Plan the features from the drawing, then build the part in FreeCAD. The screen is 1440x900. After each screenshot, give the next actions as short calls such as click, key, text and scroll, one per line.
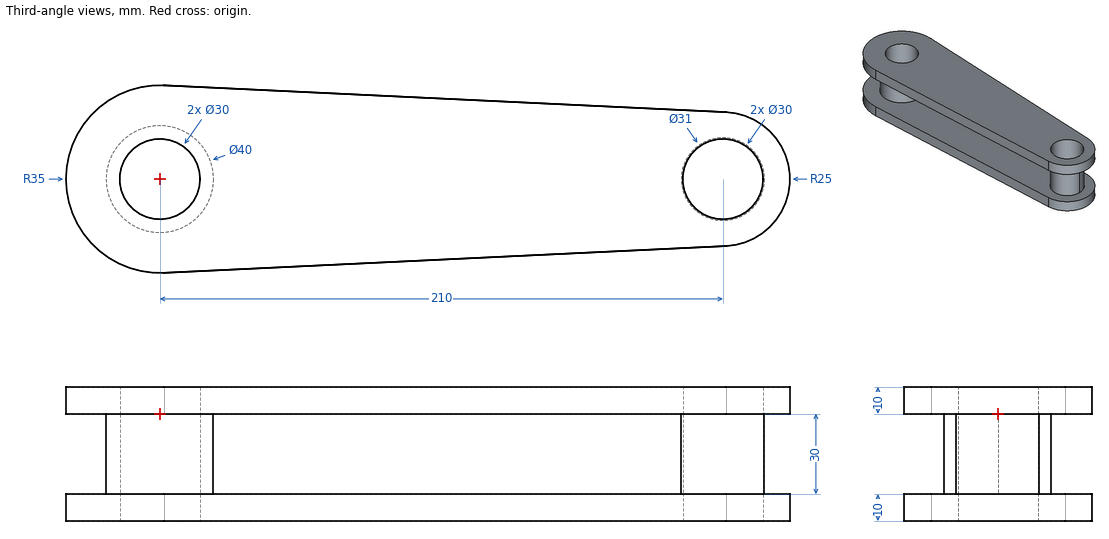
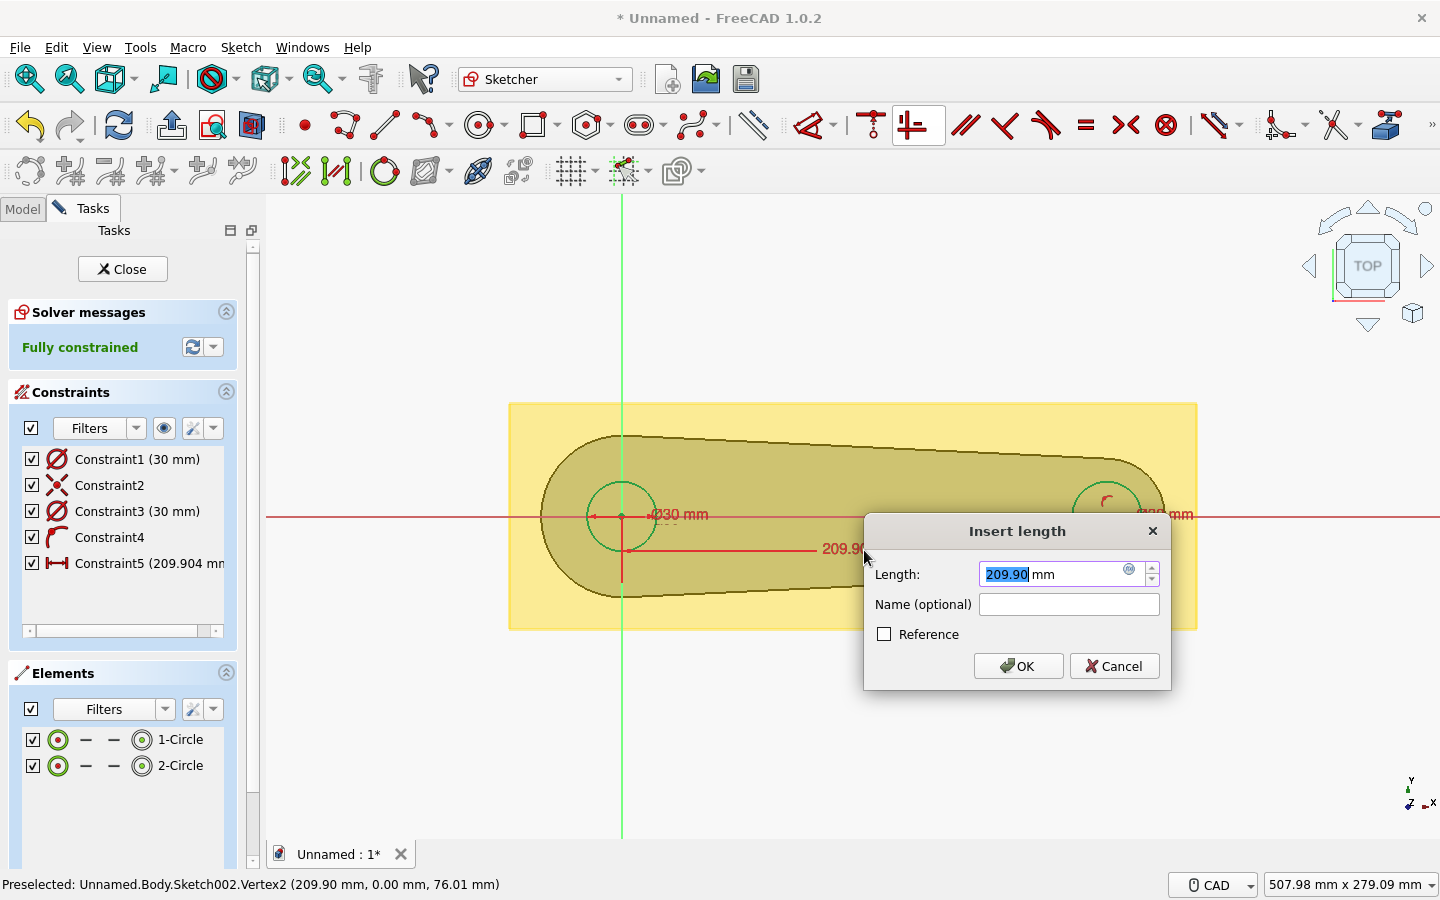
text(210)
key(Return)
key(Escape)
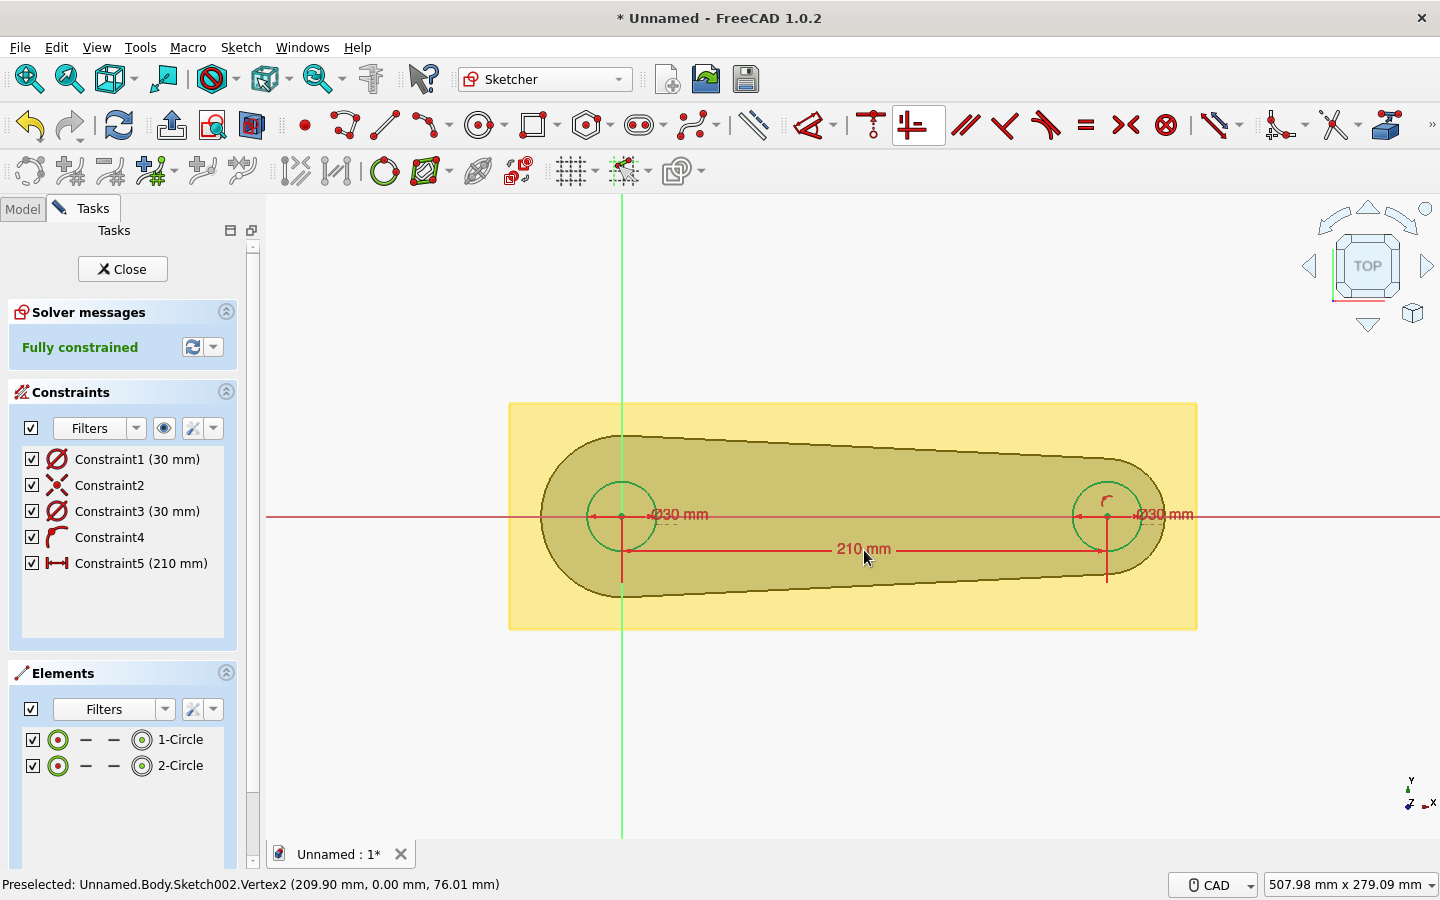
click(123, 269)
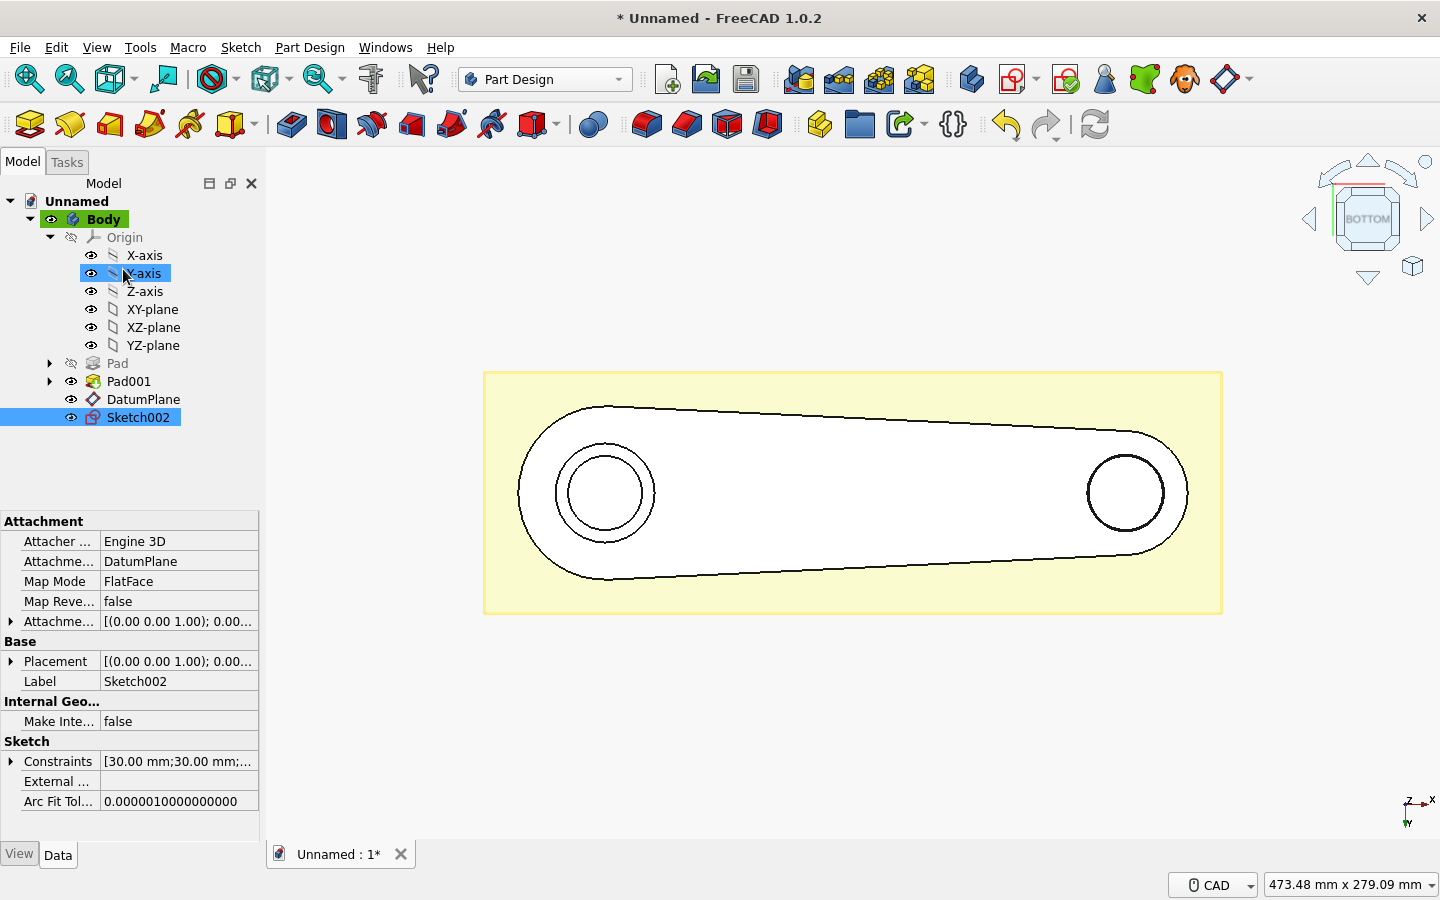
click(292, 124)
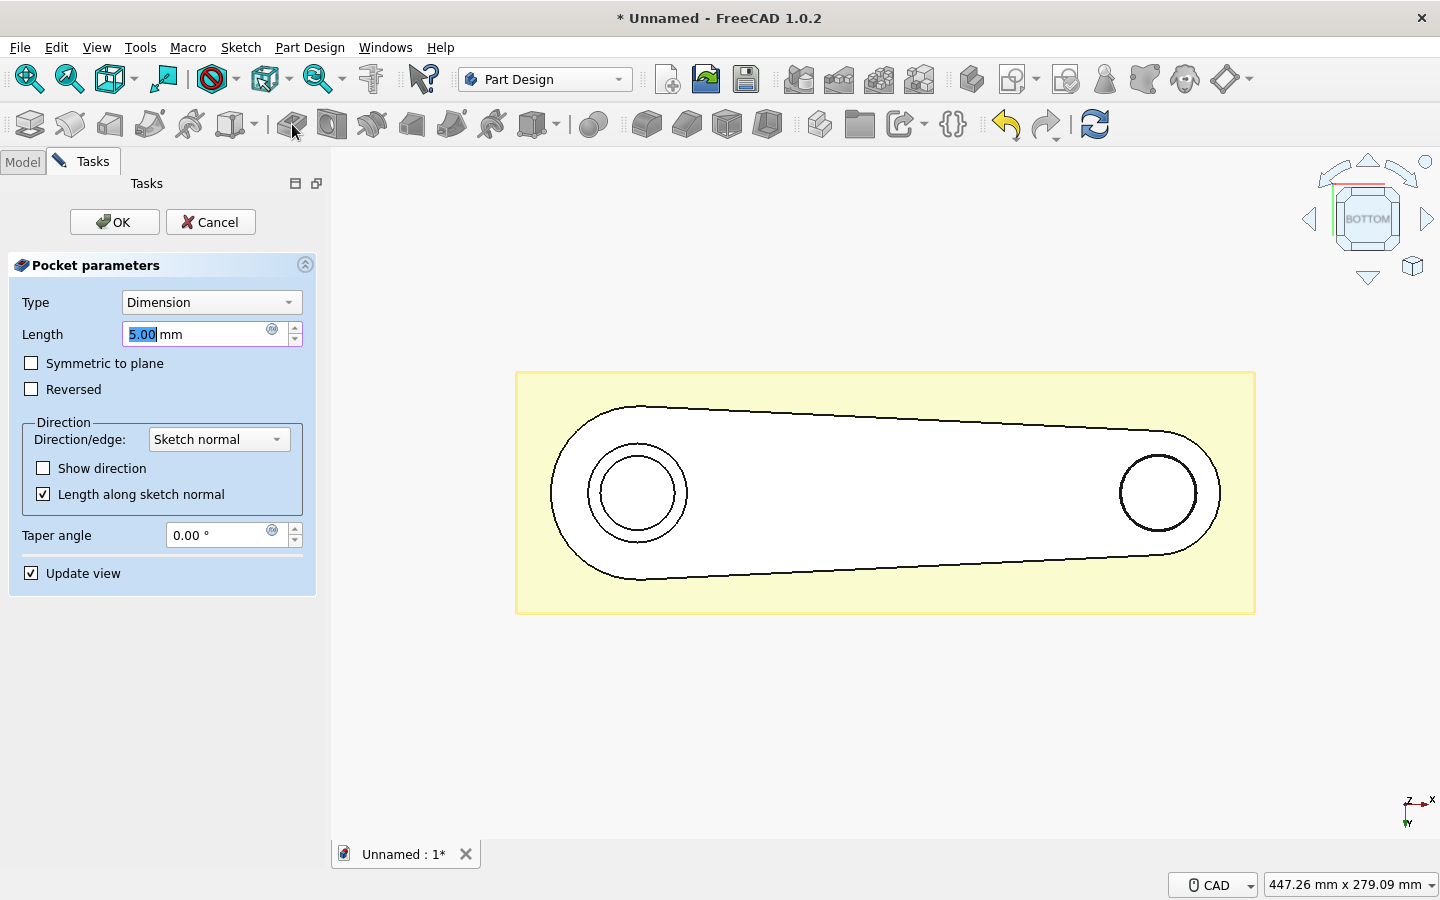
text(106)
key(Tab)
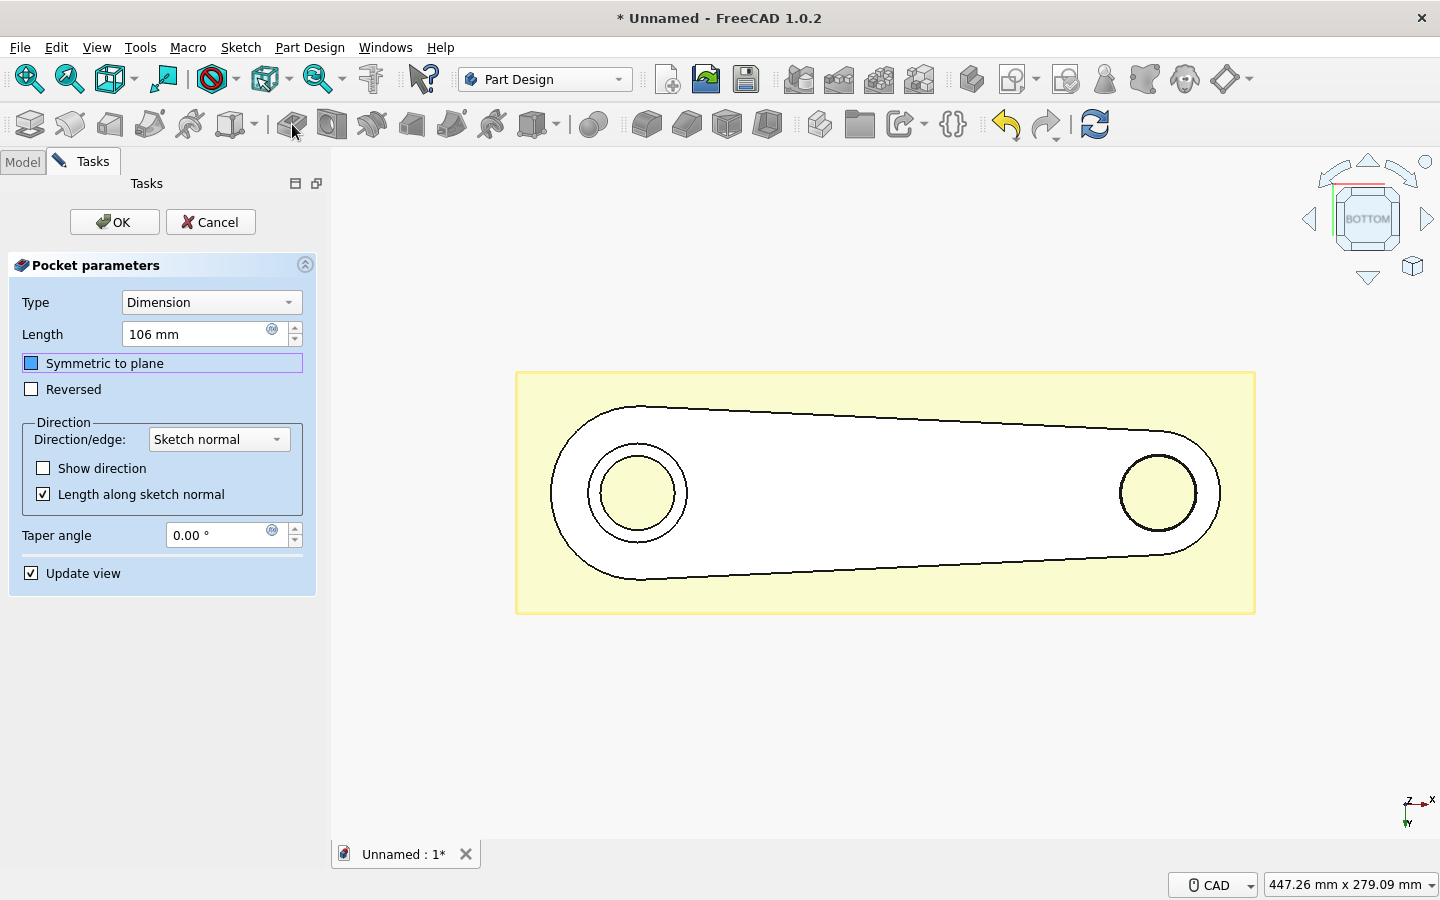
click(115, 222)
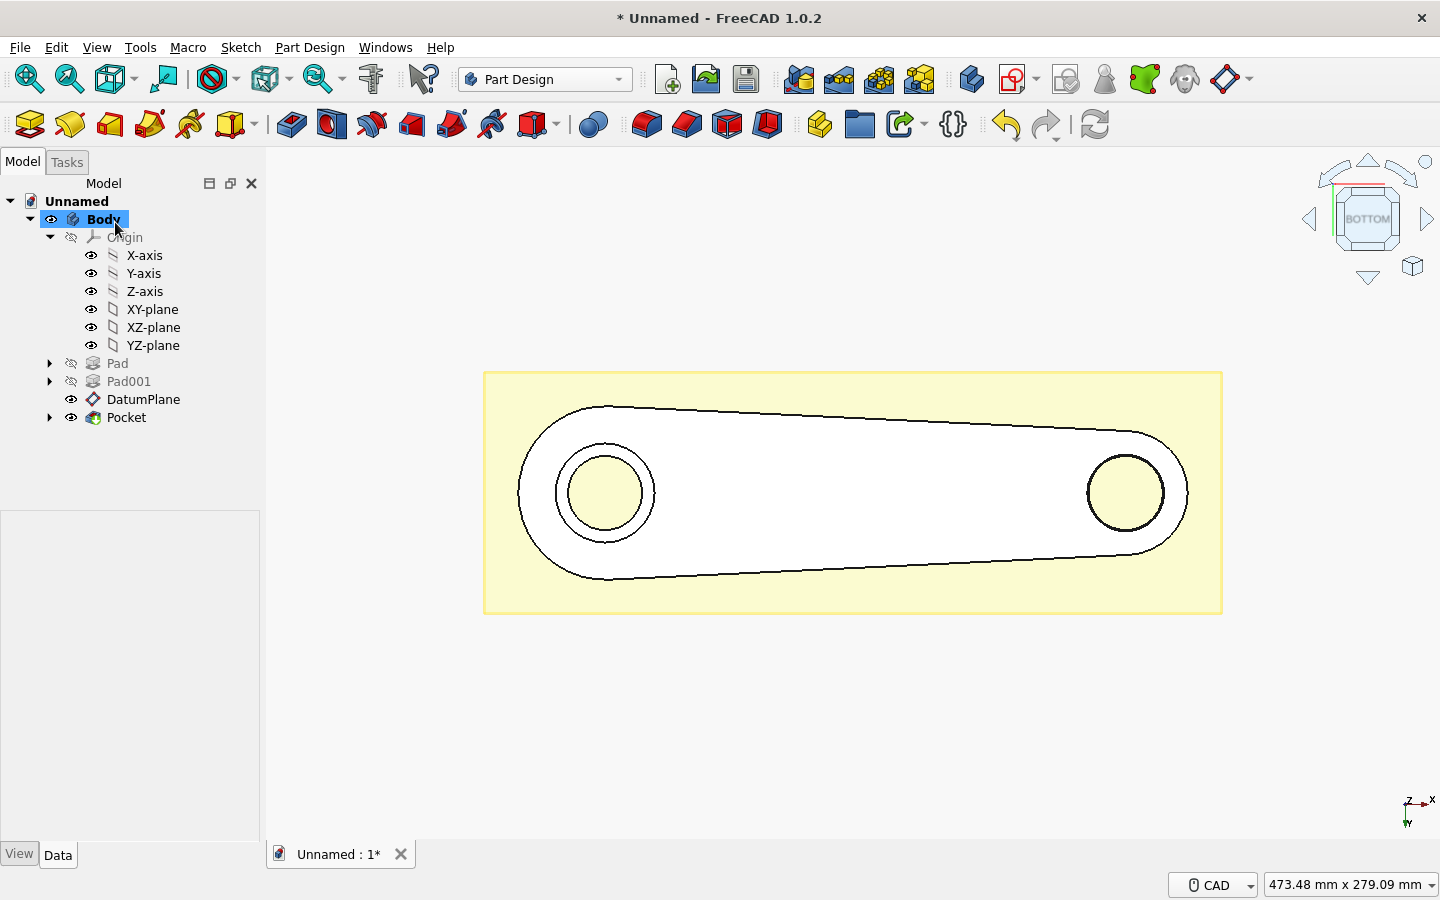
click(116, 399)
key(space)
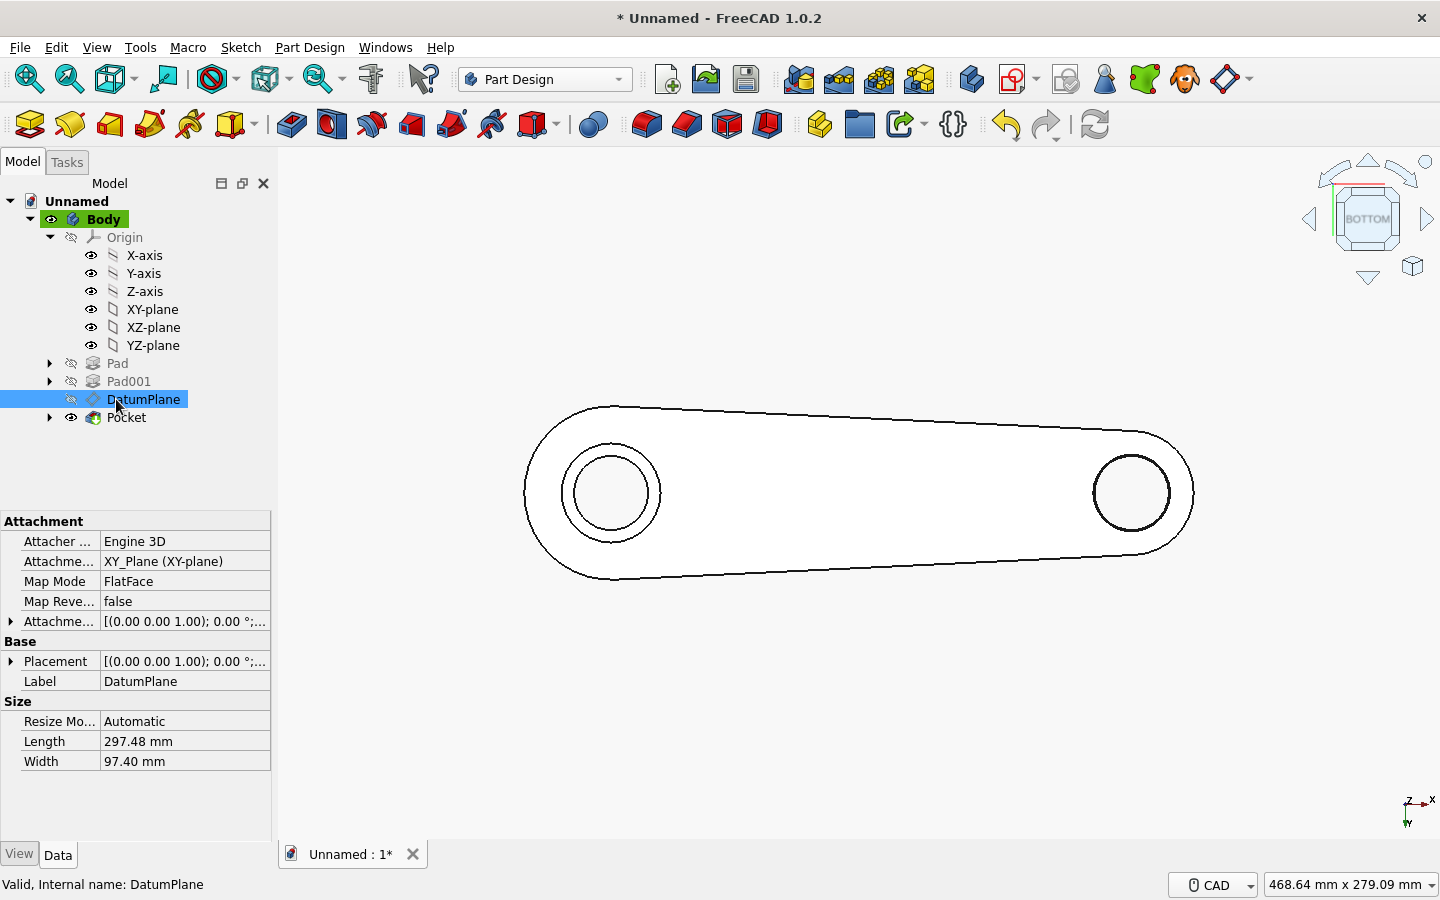
click(318, 799)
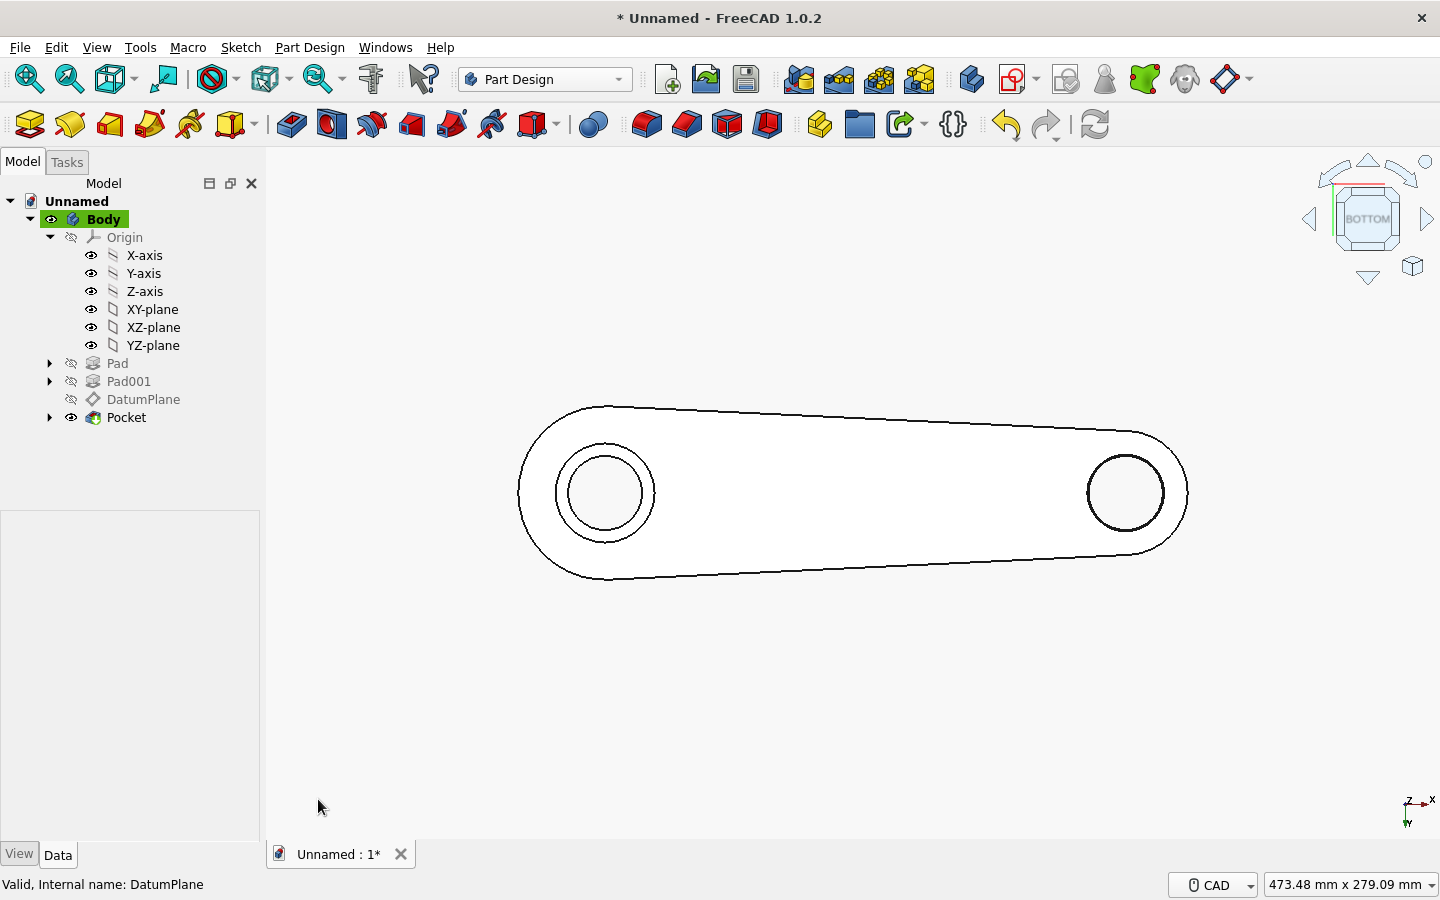
click(972, 80)